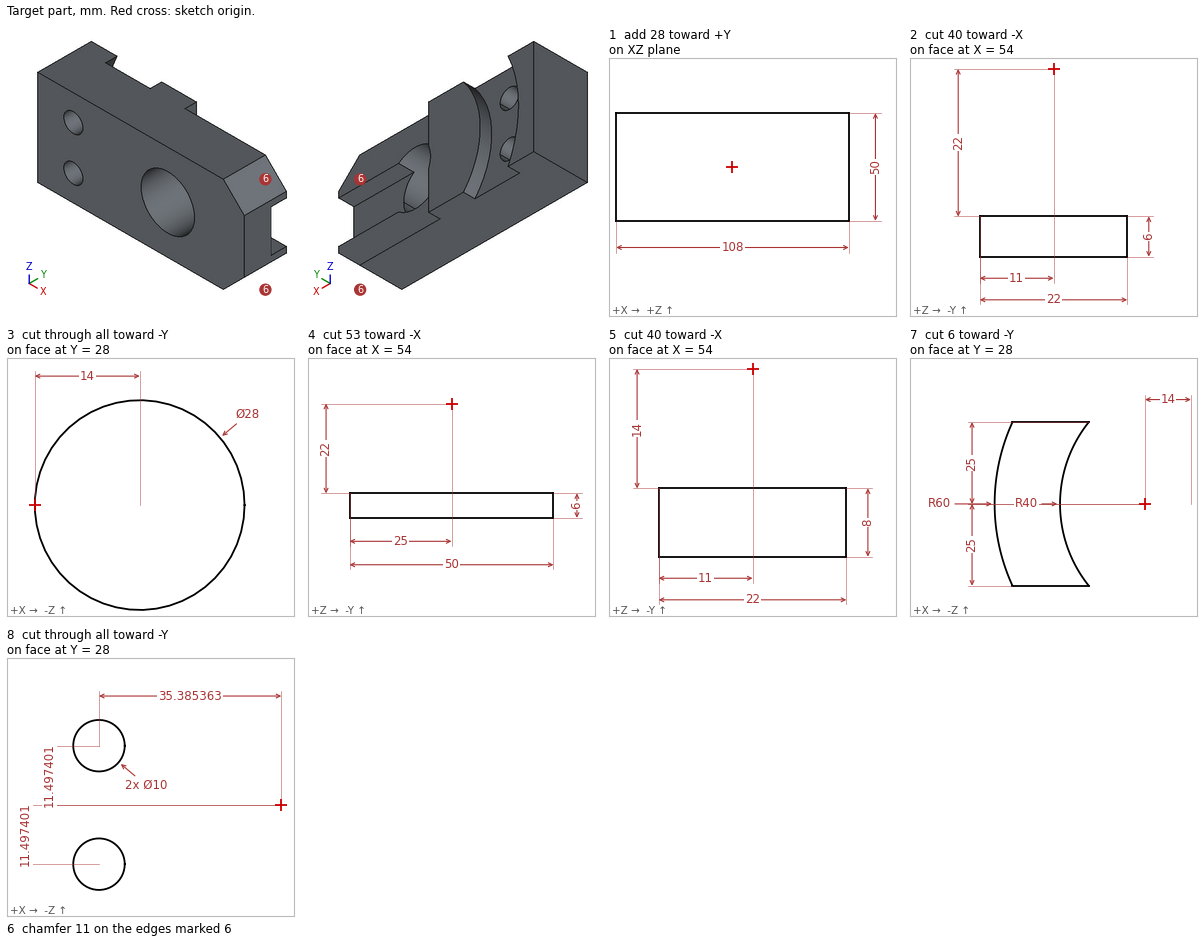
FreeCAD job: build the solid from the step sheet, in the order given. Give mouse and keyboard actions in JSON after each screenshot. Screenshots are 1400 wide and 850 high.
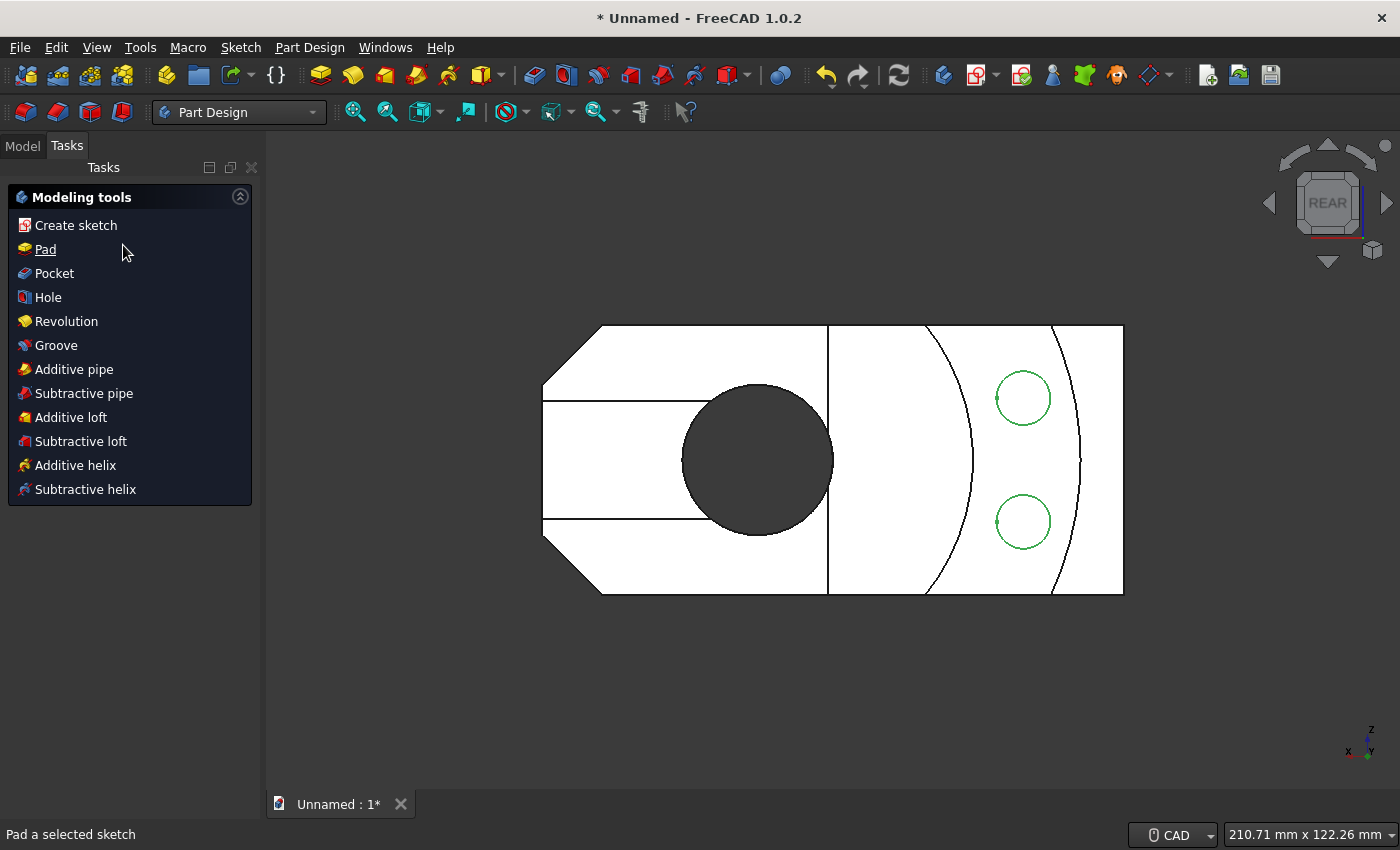
{"action": "left_click", "coordinate": [536, 76]}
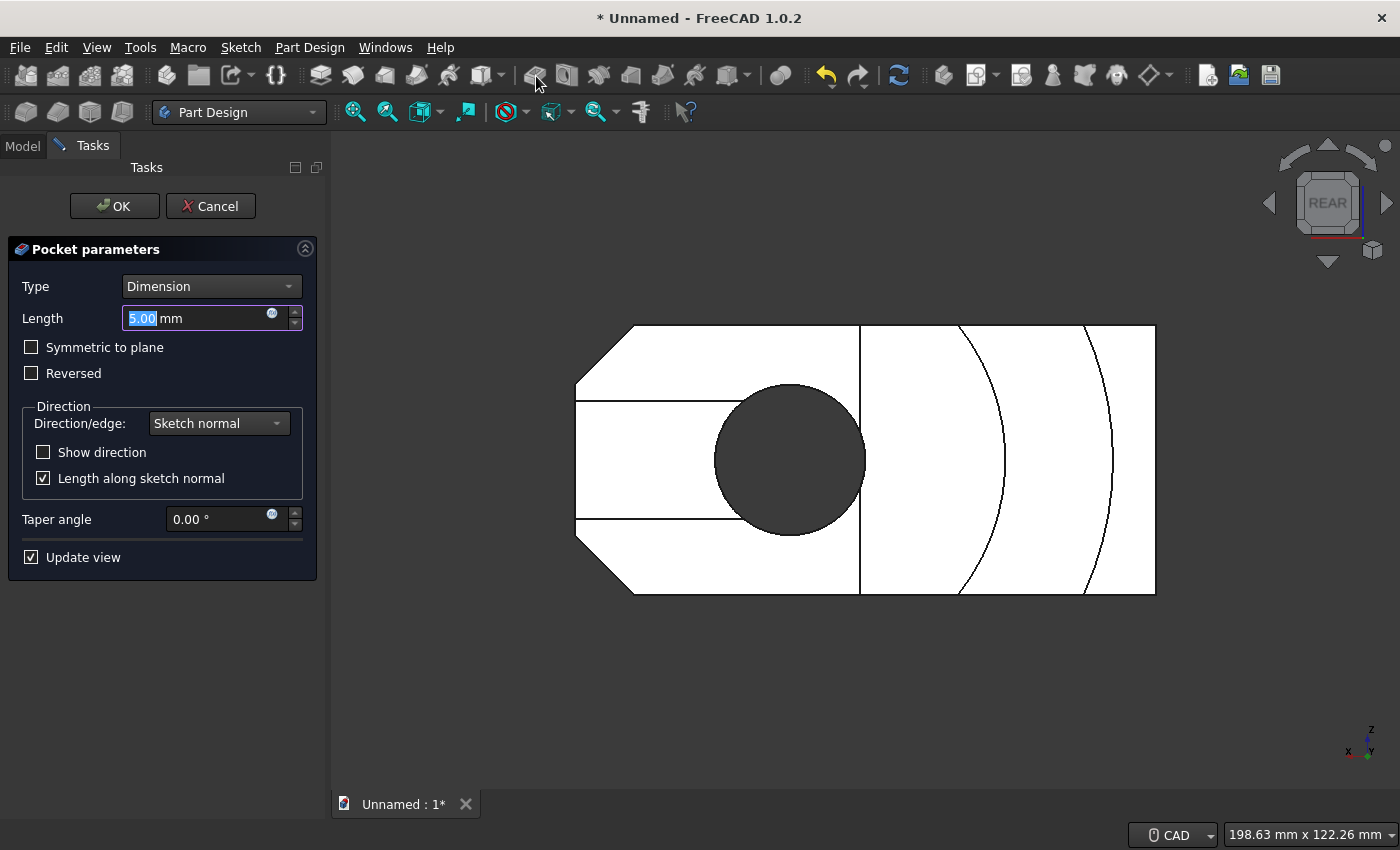
{"action": "left_click", "coordinate": [212, 286]}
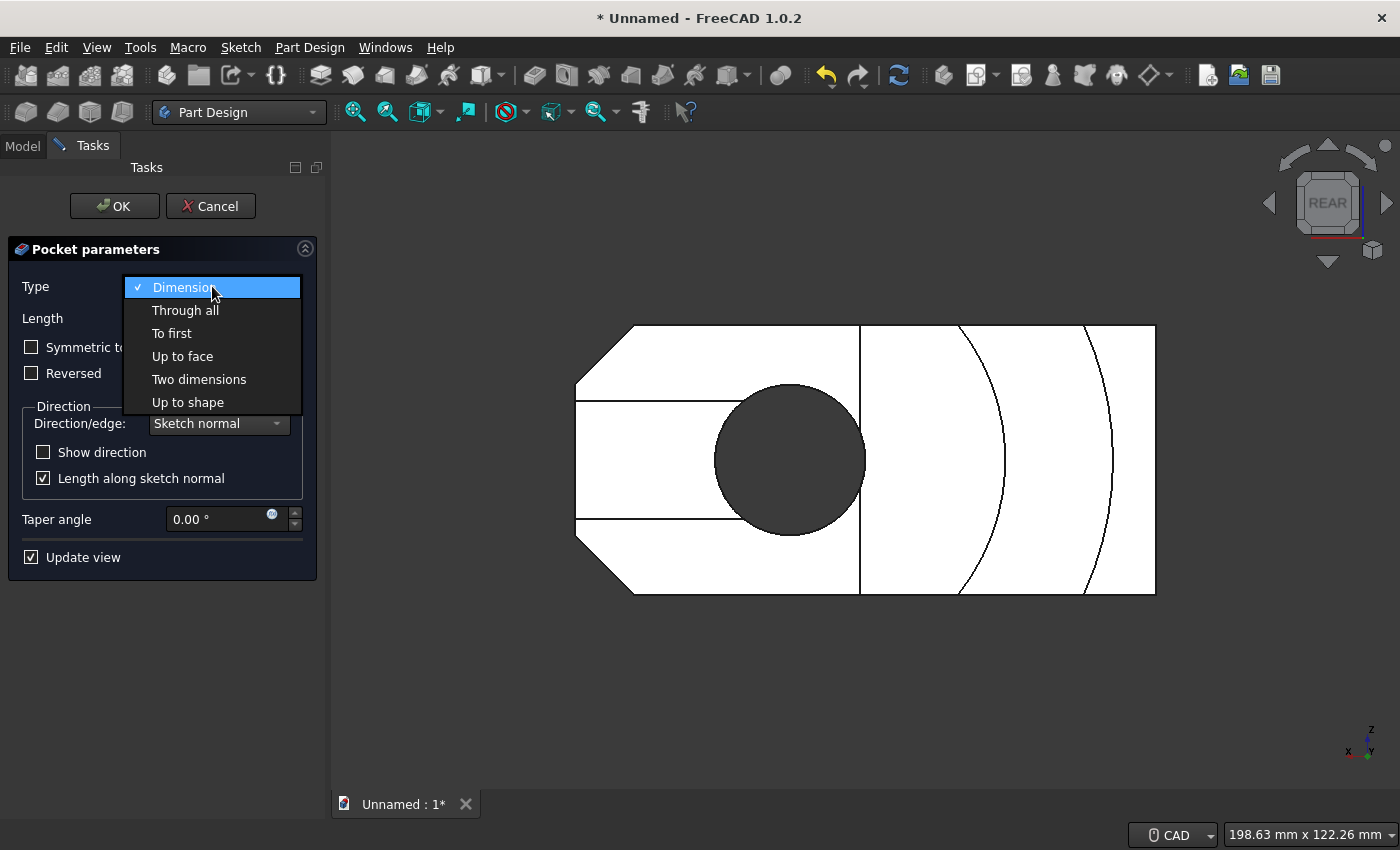
{"action": "left_click", "coordinate": [212, 310]}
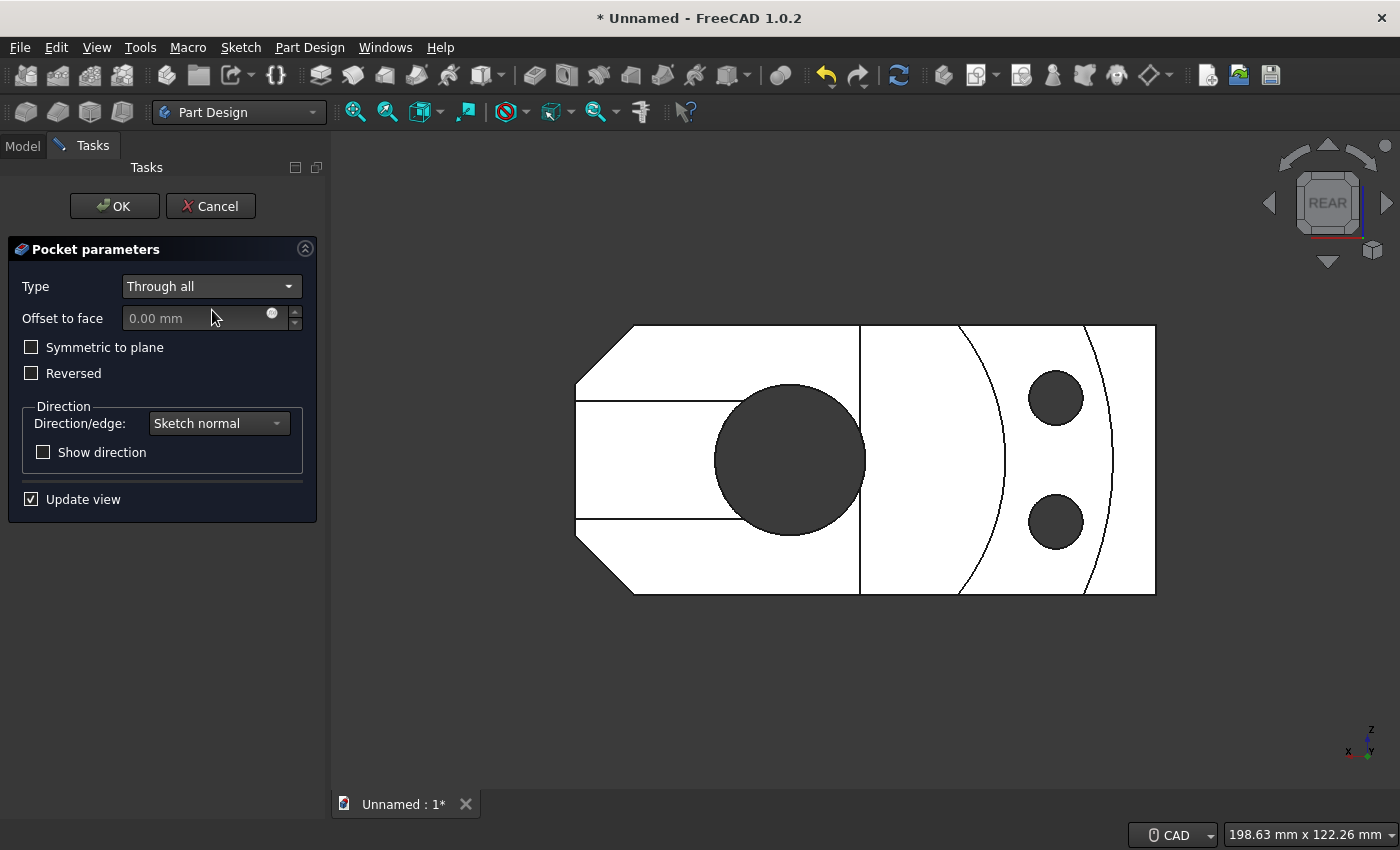
{"action": "left_click", "coordinate": [115, 206]}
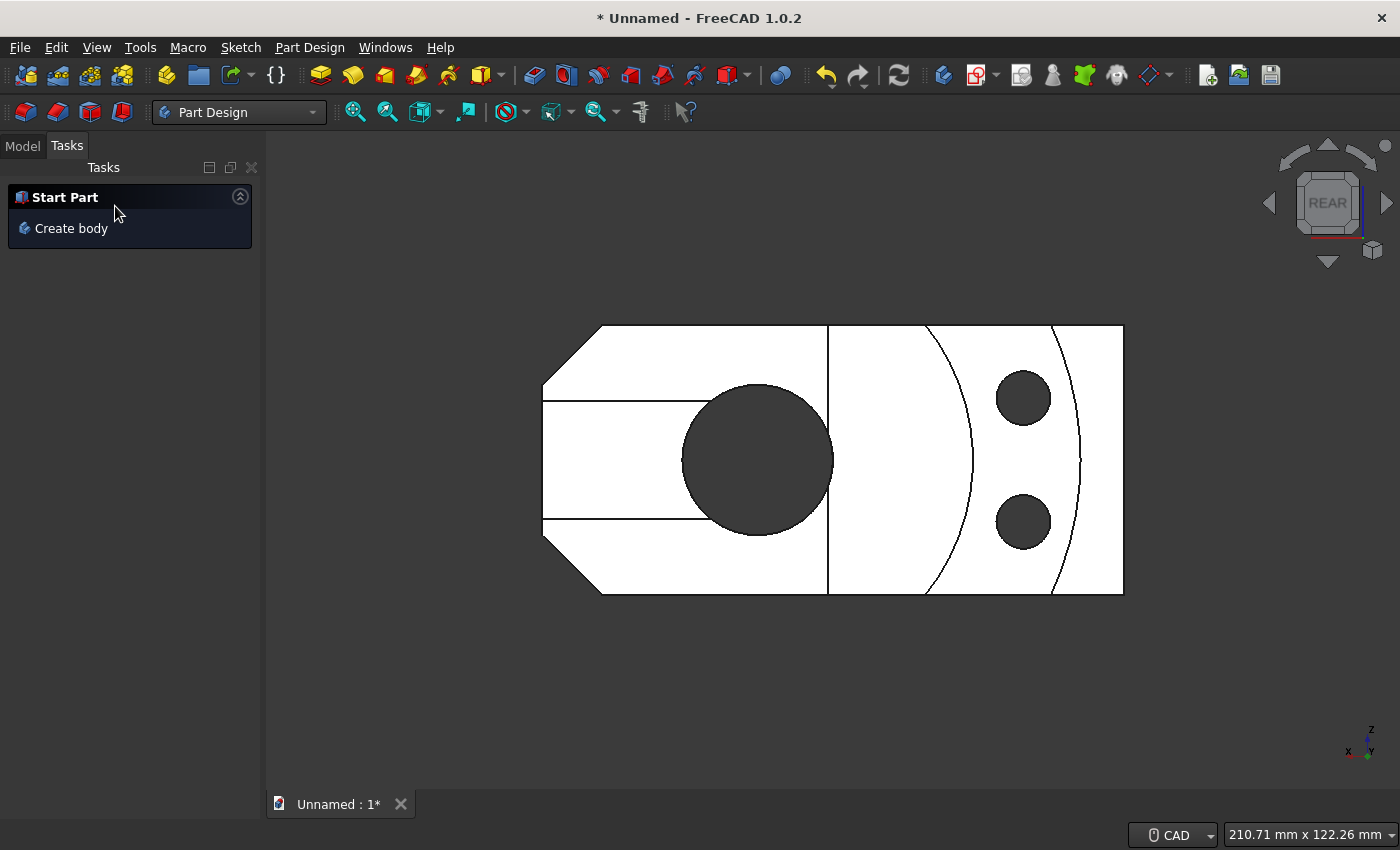
{"action": "key", "text": "0"}